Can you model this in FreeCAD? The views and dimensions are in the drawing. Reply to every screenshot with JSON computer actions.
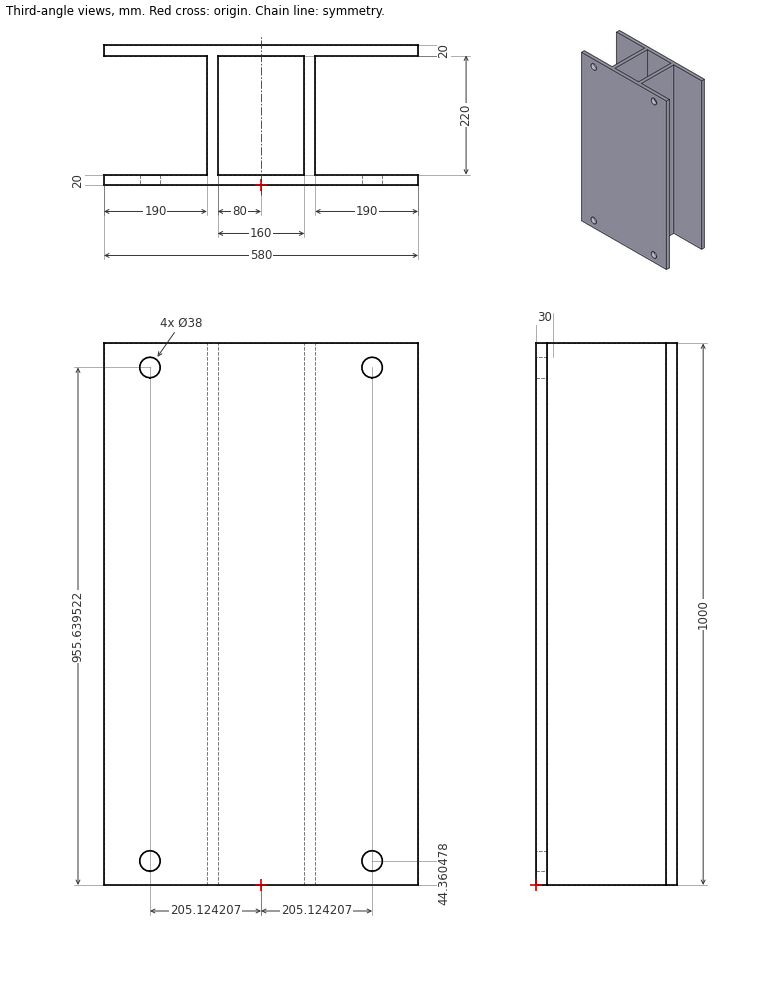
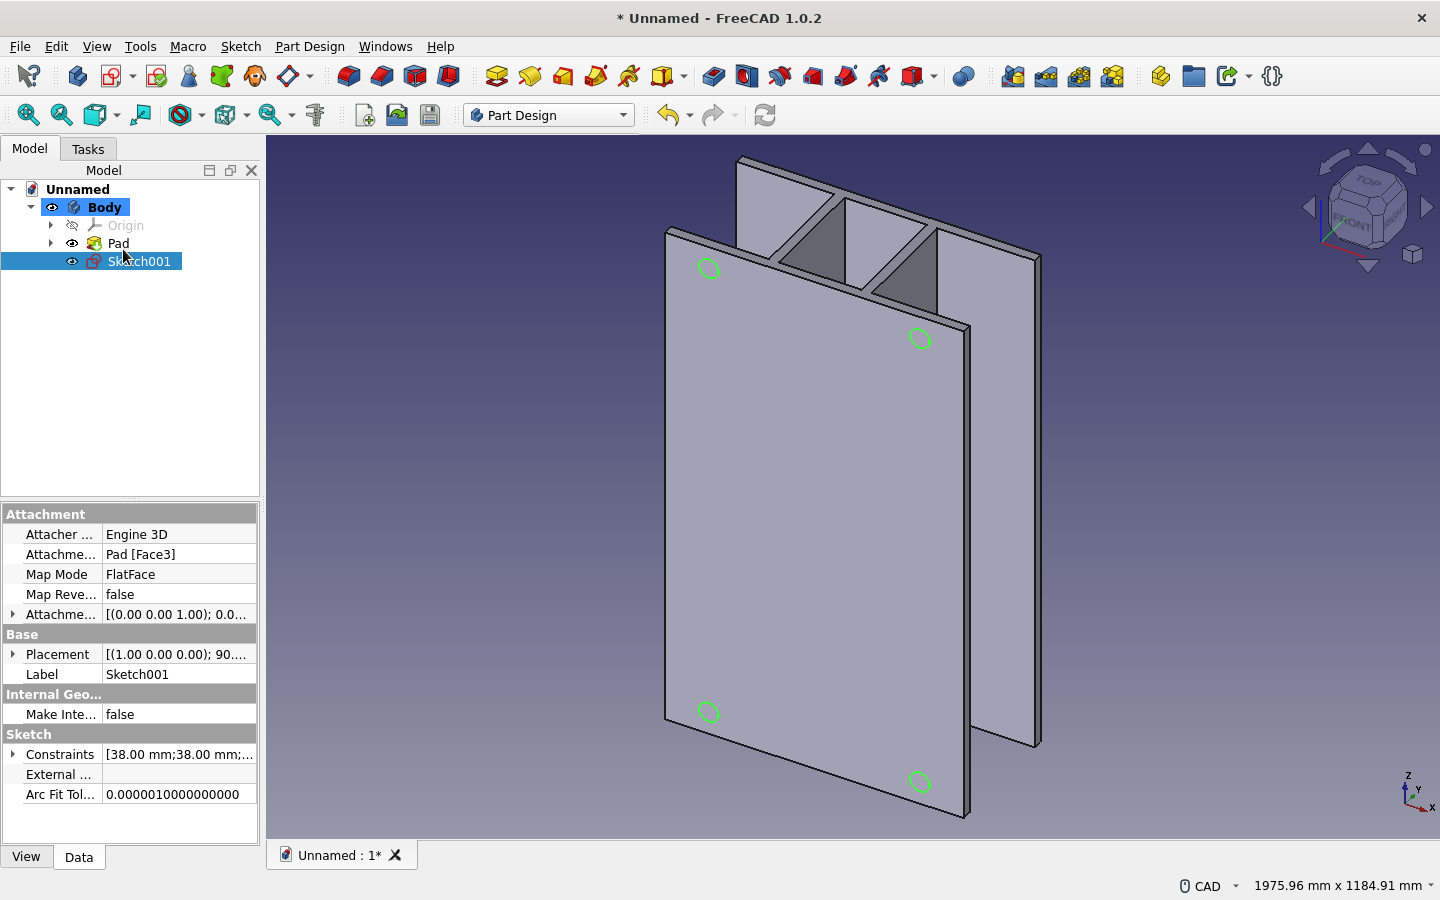
{"action": "left_click", "coordinate": [714, 76]}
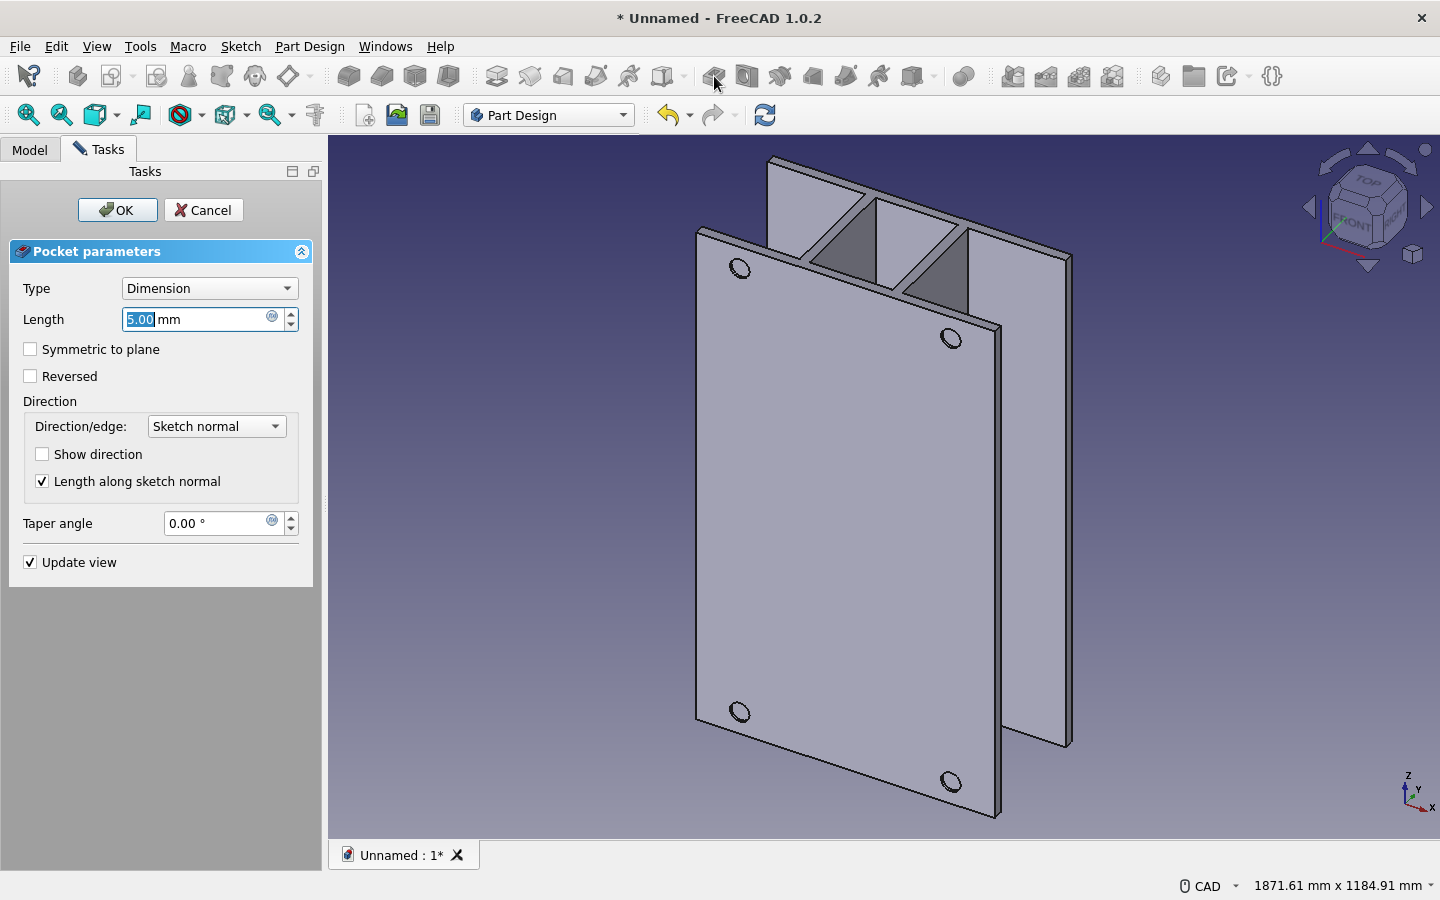
{"action": "type", "text": "30"}
{"action": "key", "text": "Tab"}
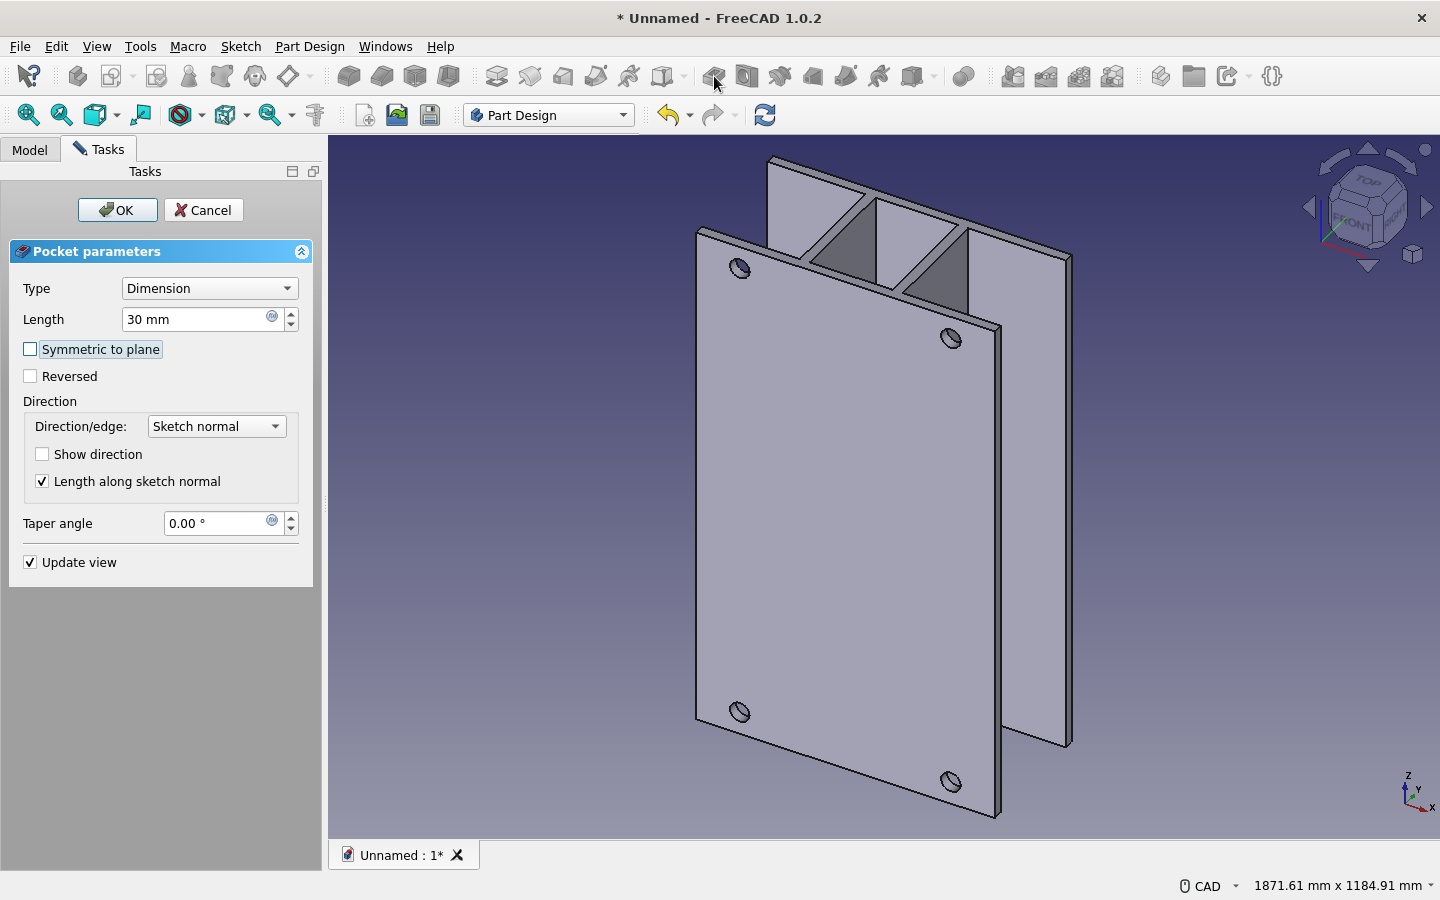
{"action": "left_click", "coordinate": [118, 210]}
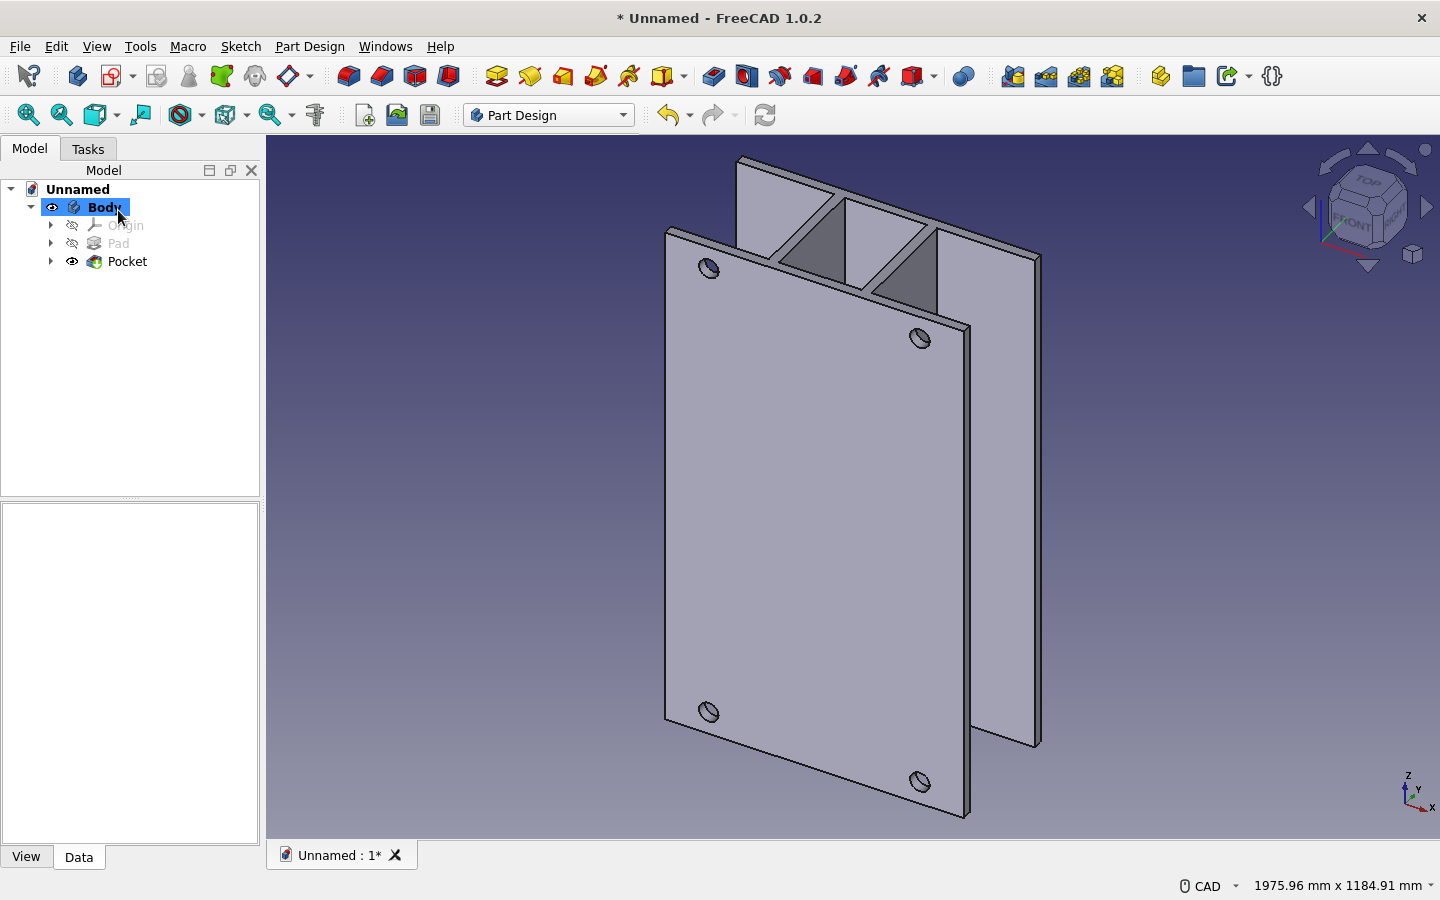
{"action": "key", "text": "0"}